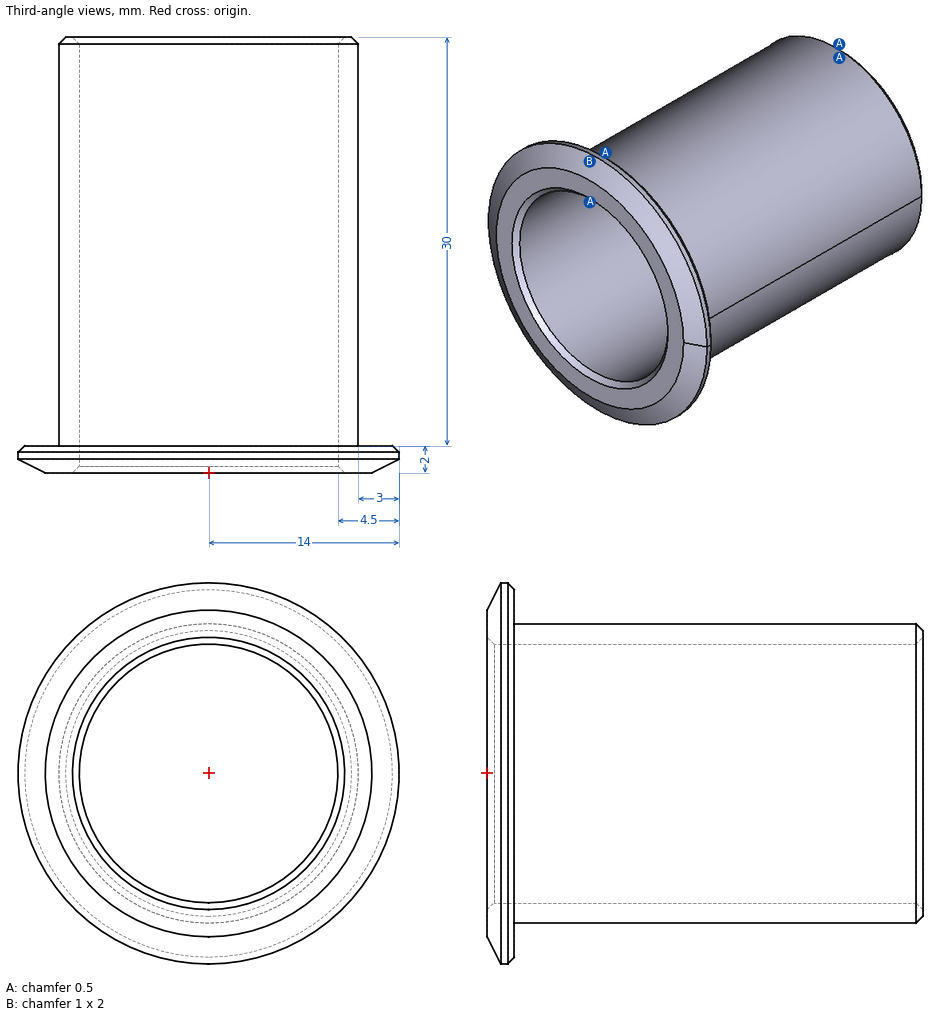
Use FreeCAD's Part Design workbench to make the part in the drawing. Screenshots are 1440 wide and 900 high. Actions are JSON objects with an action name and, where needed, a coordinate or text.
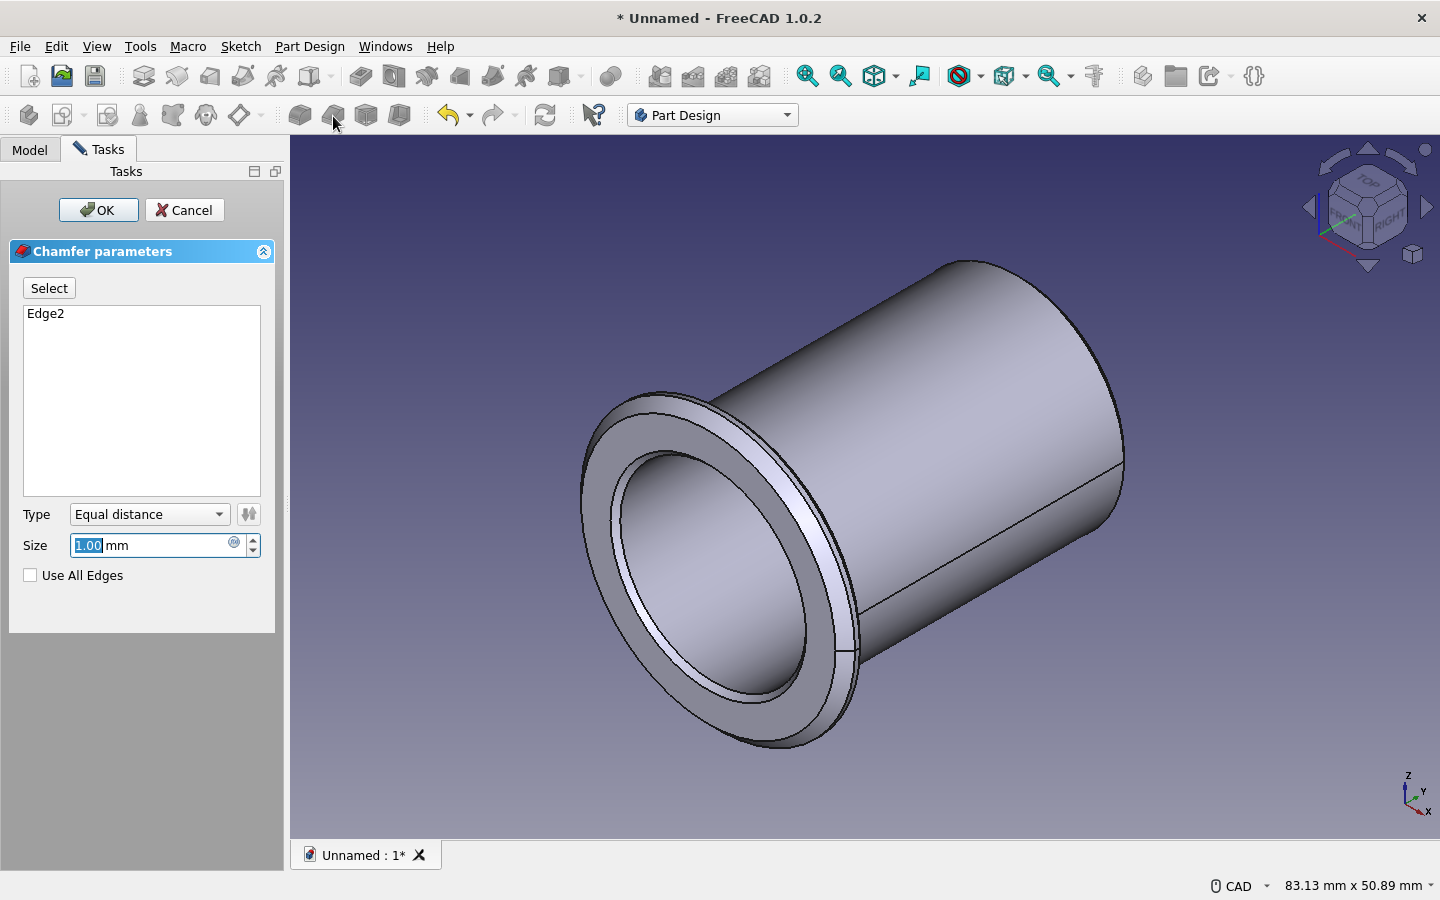
{"action": "type", "text": "1"}
{"action": "key", "text": "Tab"}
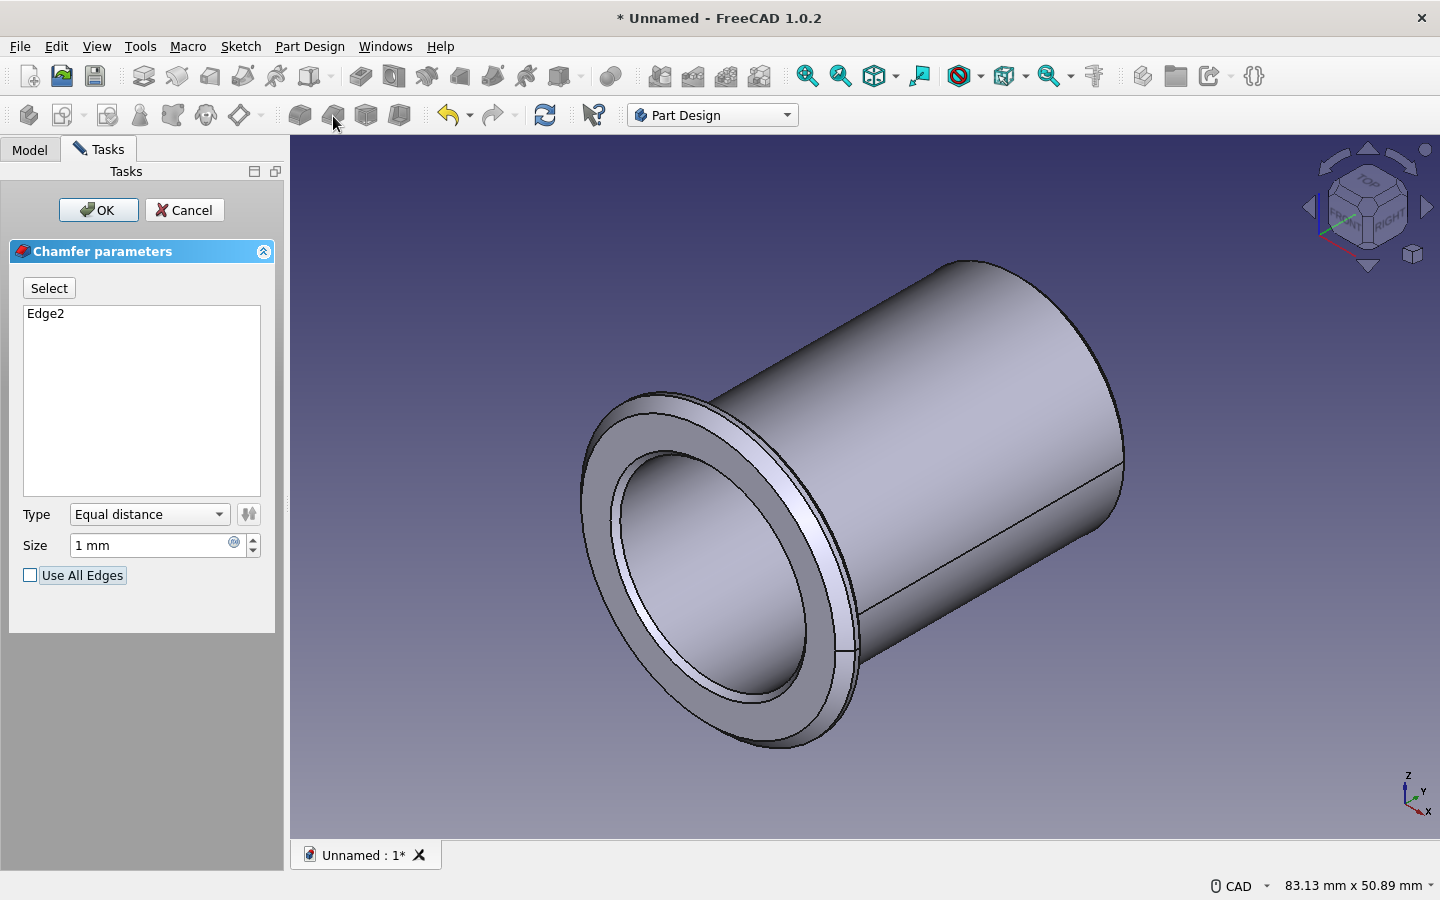
{"action": "left_click", "coordinate": [150, 514]}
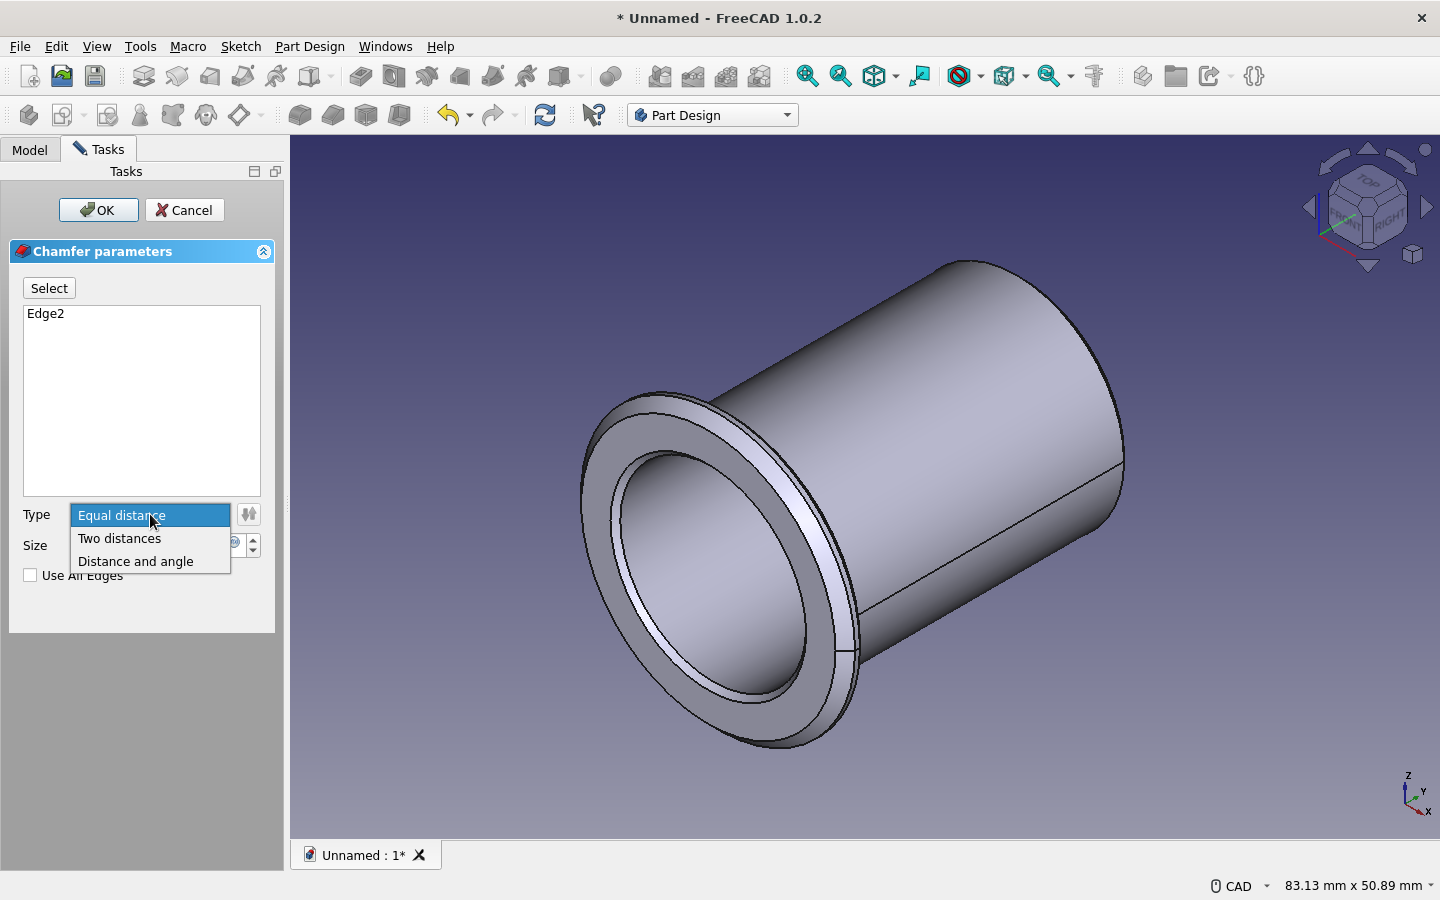
{"action": "left_click", "coordinate": [148, 538]}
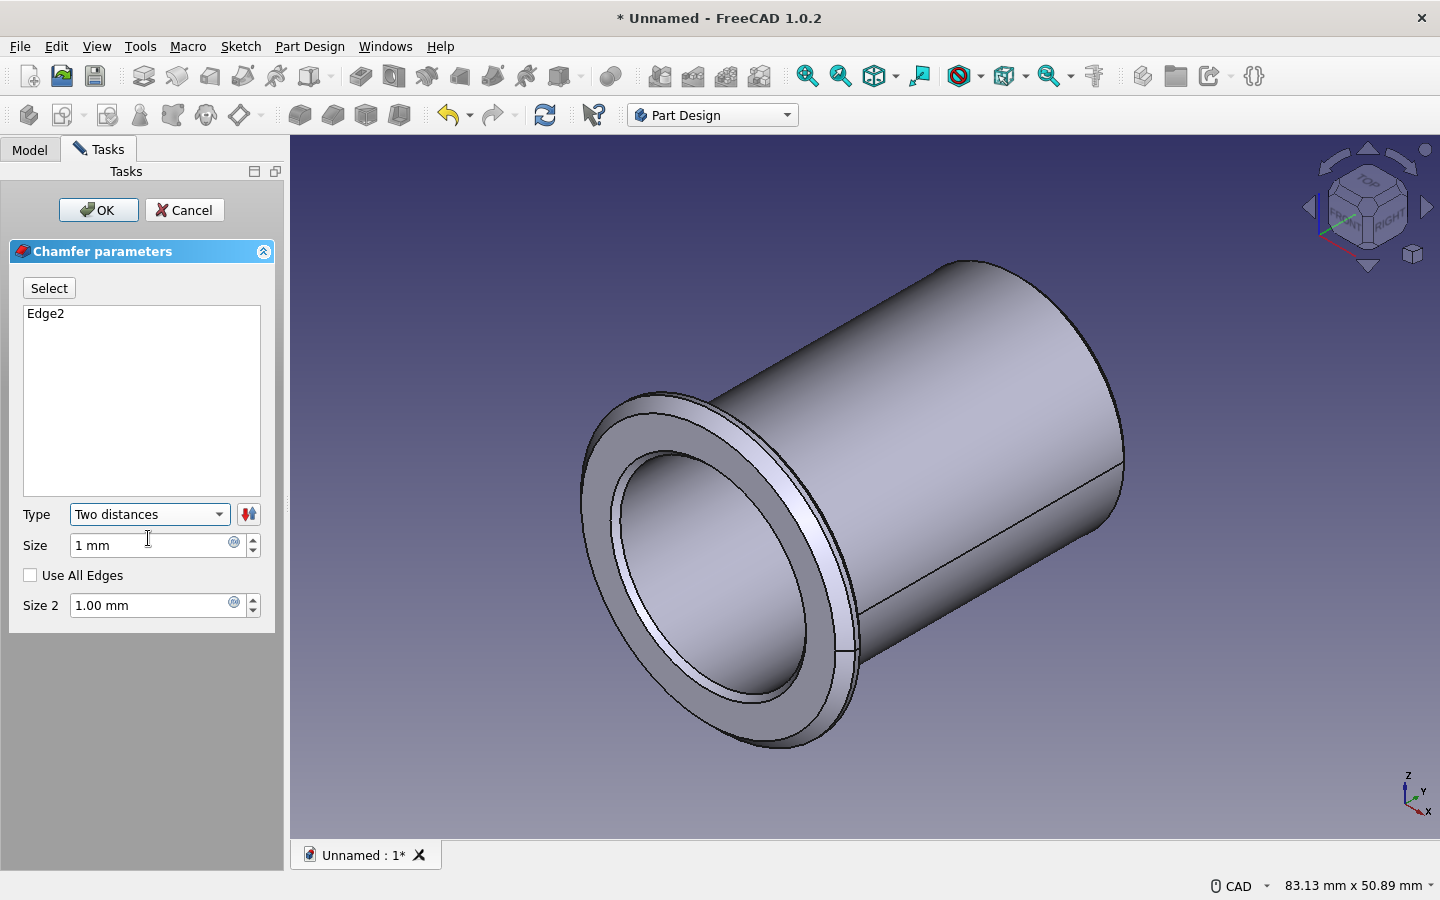
{"action": "triple_click", "coordinate": [158, 606]}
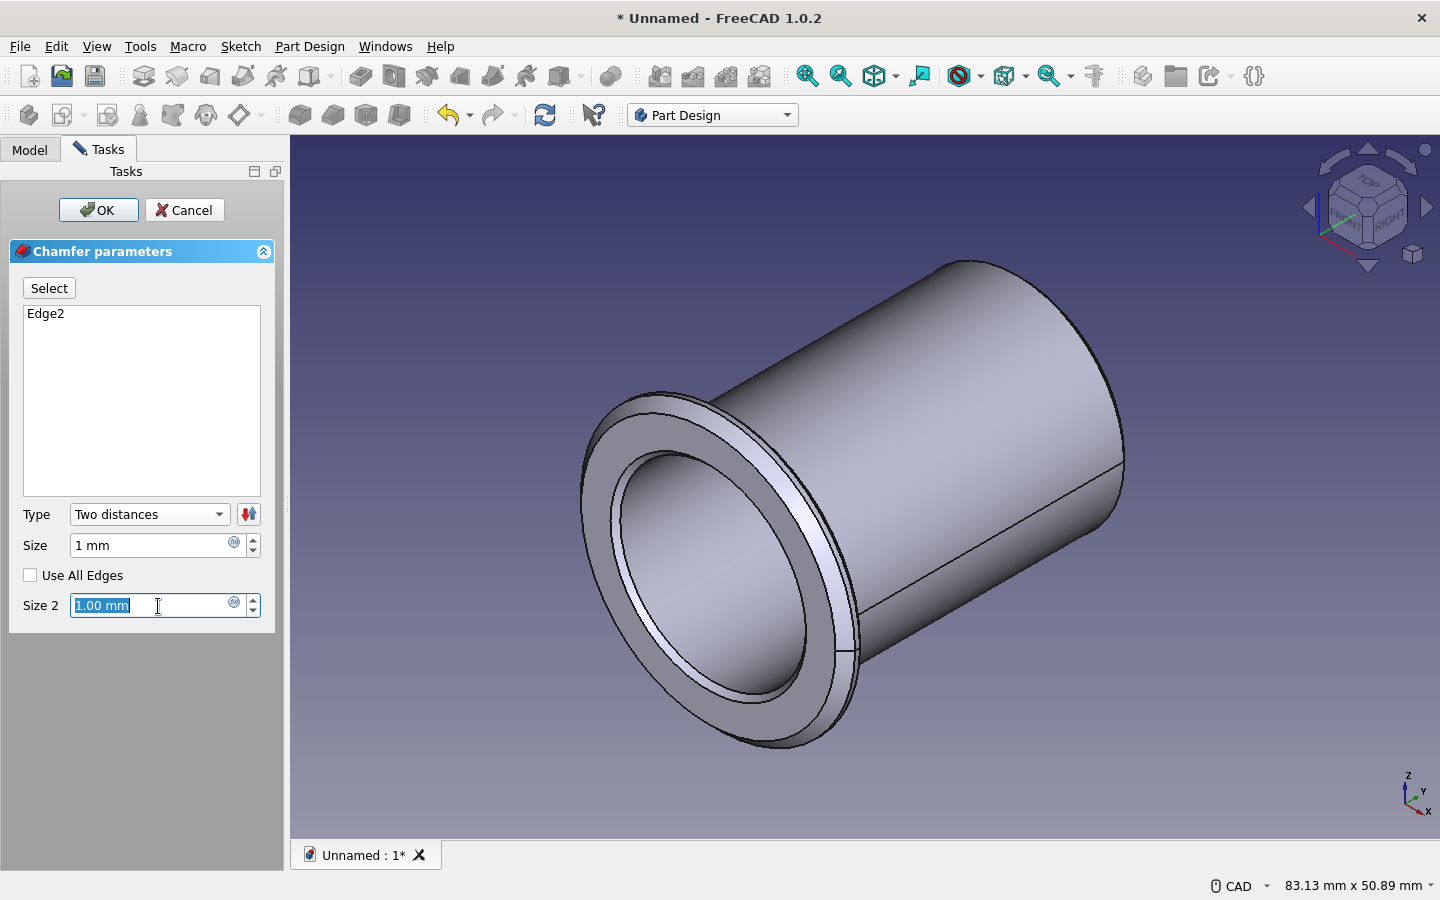
{"action": "type", "text": "2"}
{"action": "key", "text": "Tab"}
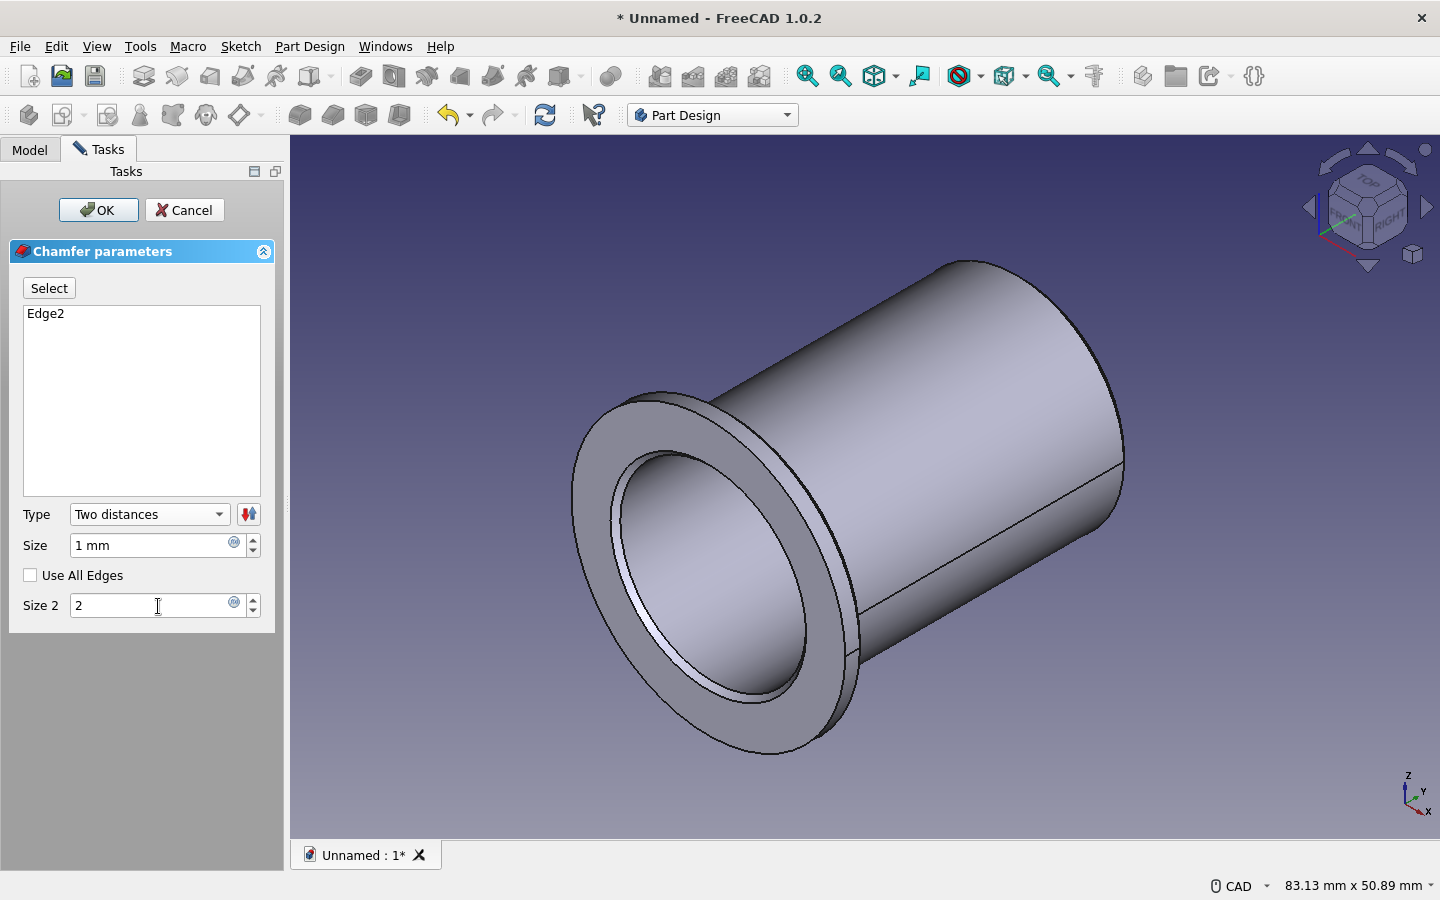
{"action": "left_click", "coordinate": [249, 514]}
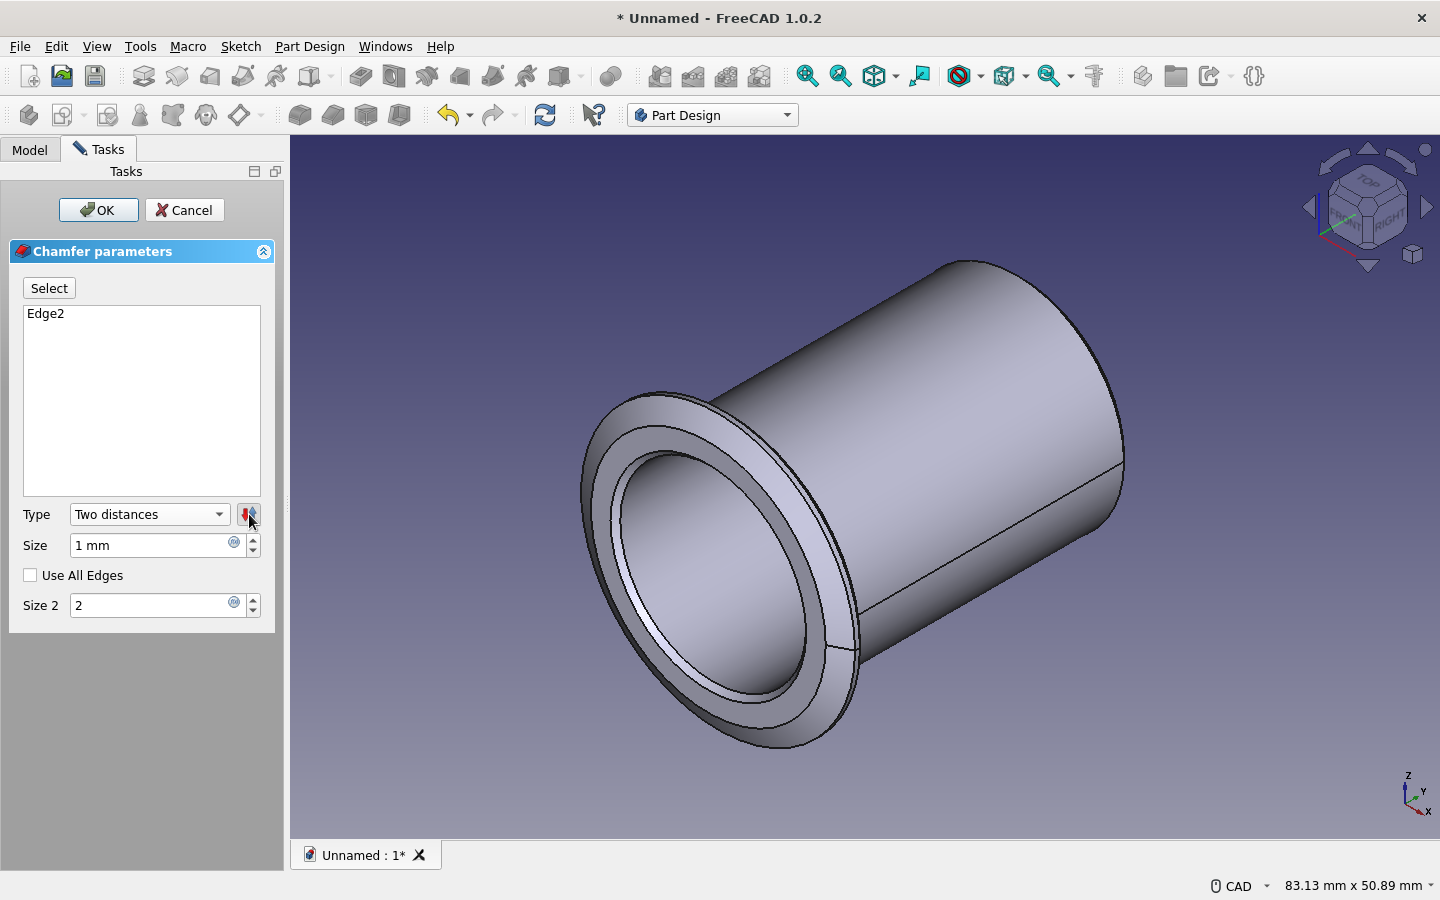
{"action": "left_click", "coordinate": [99, 210]}